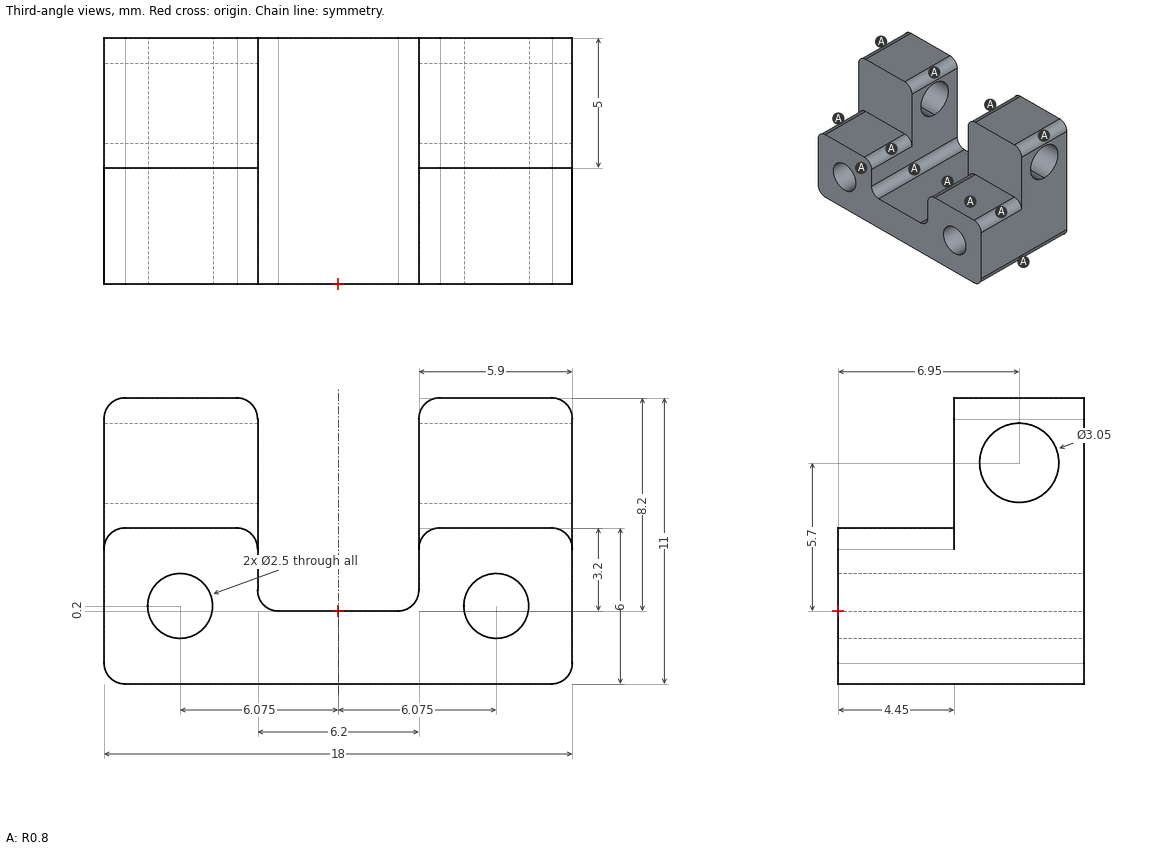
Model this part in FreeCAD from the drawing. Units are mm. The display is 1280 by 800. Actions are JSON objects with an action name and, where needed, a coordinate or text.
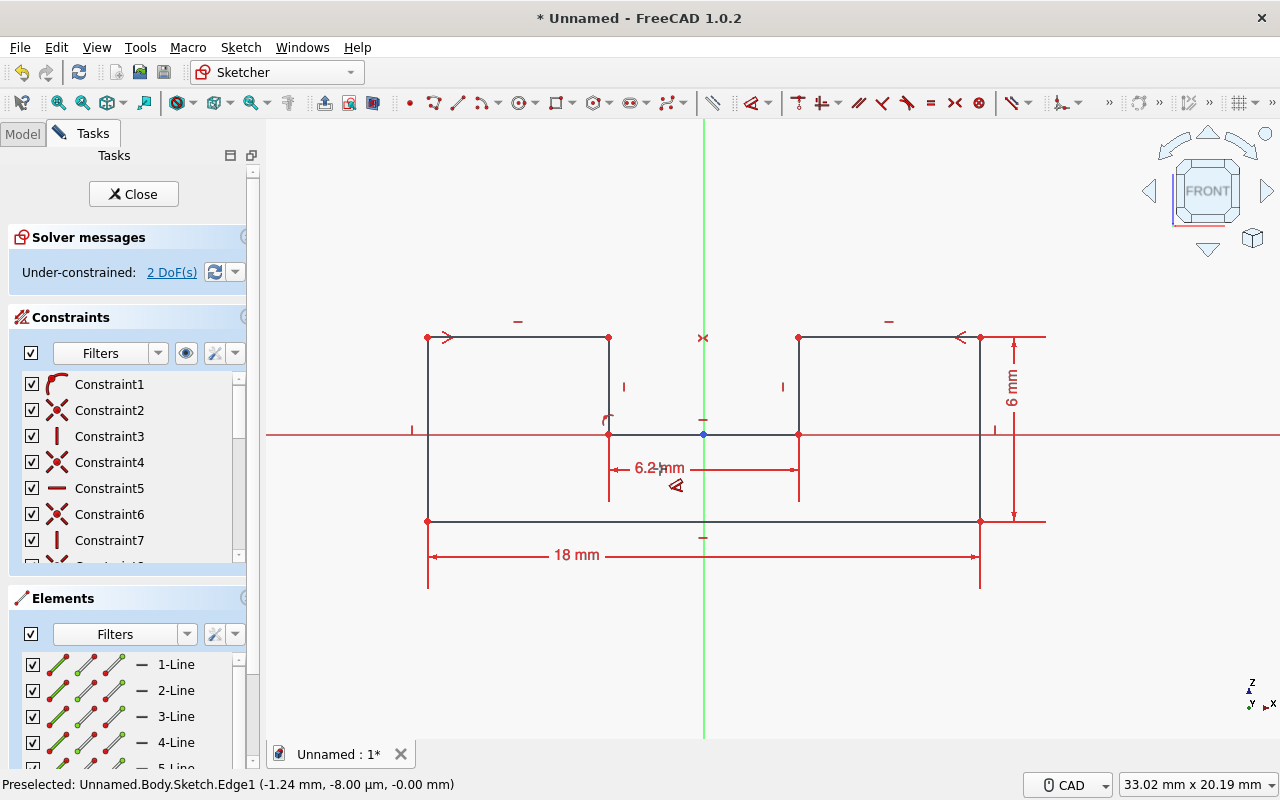
{"action": "left_click", "coordinate": [799, 406]}
{"action": "left_click", "coordinate": [833, 386]}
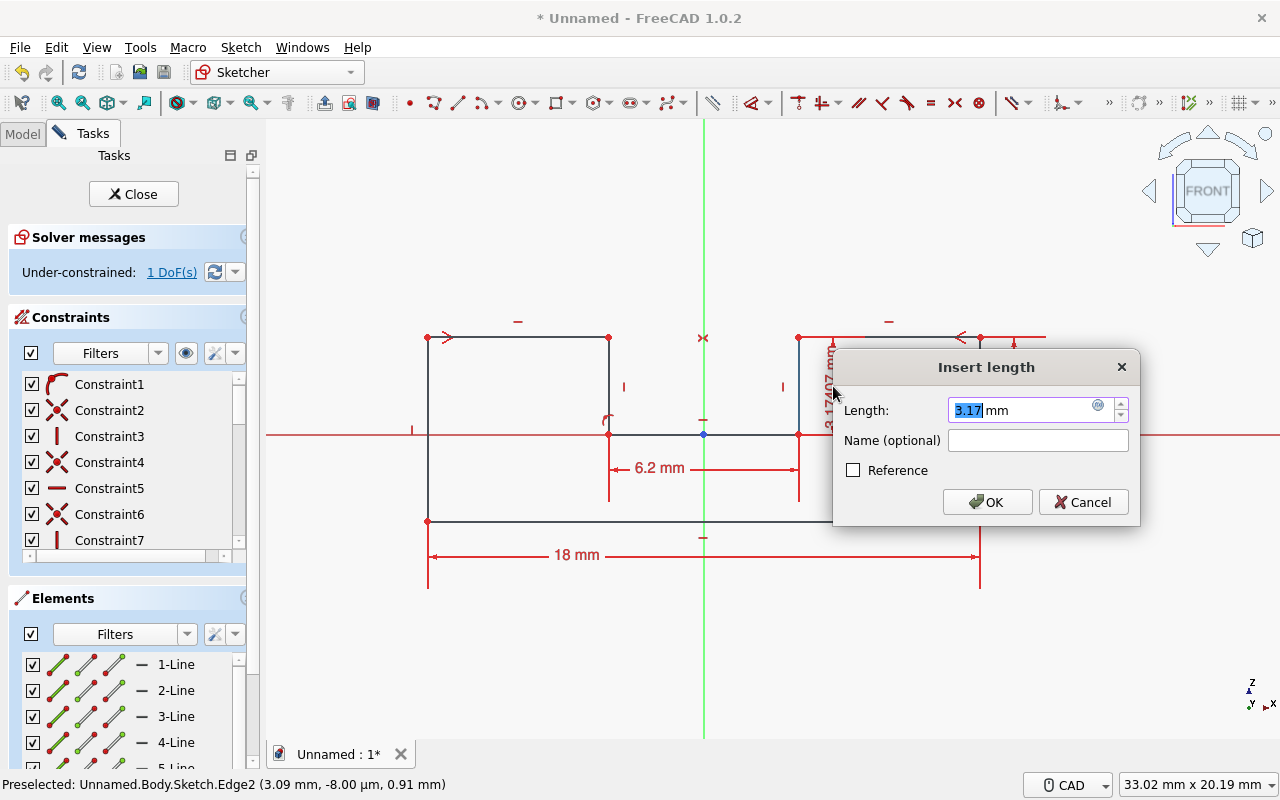
{"action": "type", "text": "3.2"}
{"action": "key", "text": "Return"}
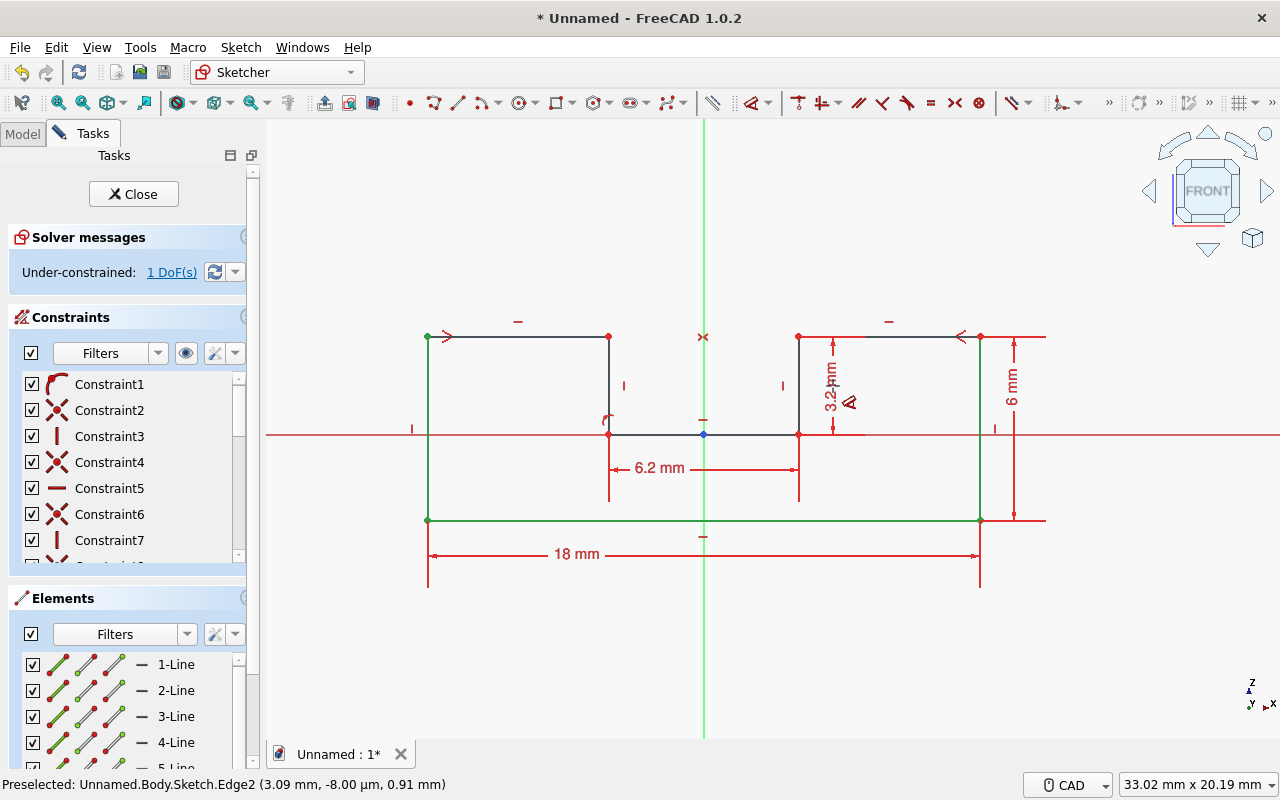
{"action": "left_click", "coordinate": [853, 337]}
{"action": "left_click", "coordinate": [890, 303]}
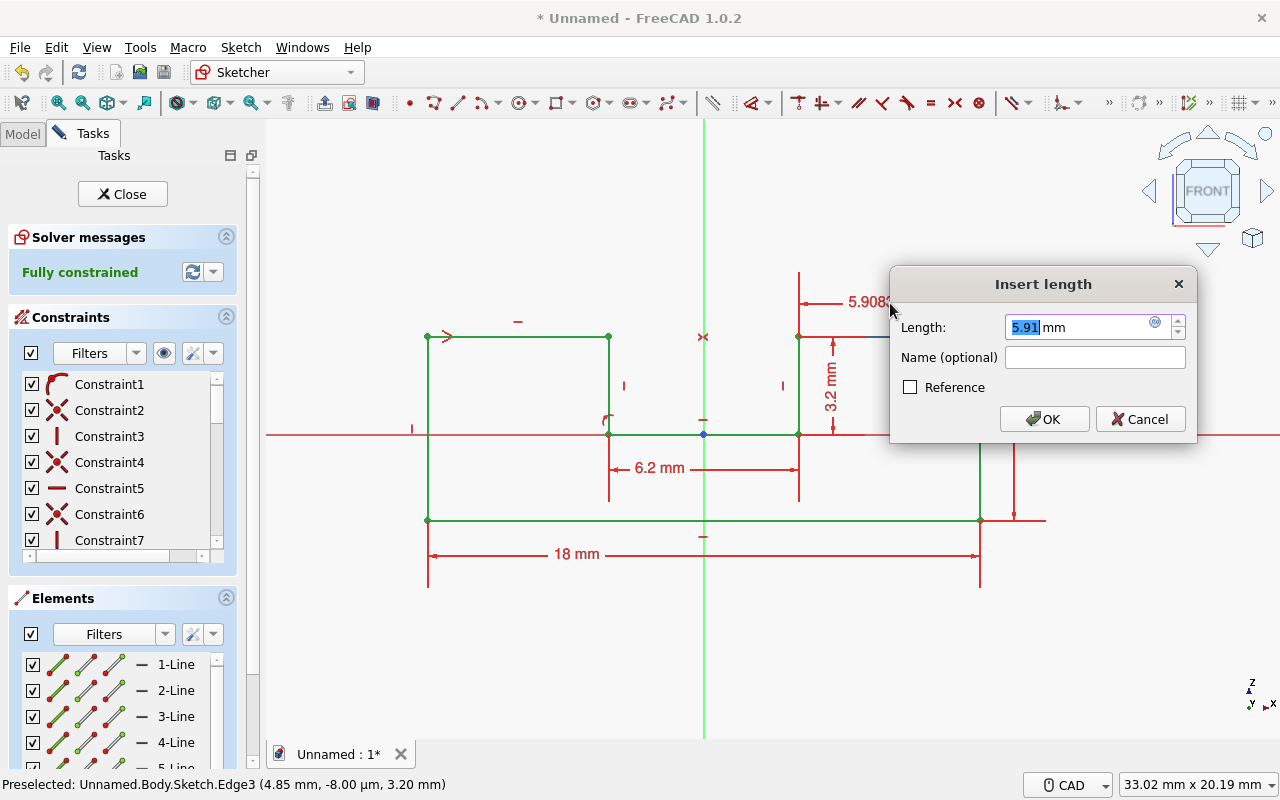
{"action": "type", "text": "5.9"}
{"action": "key", "text": "Return"}
{"action": "key", "text": "Escape"}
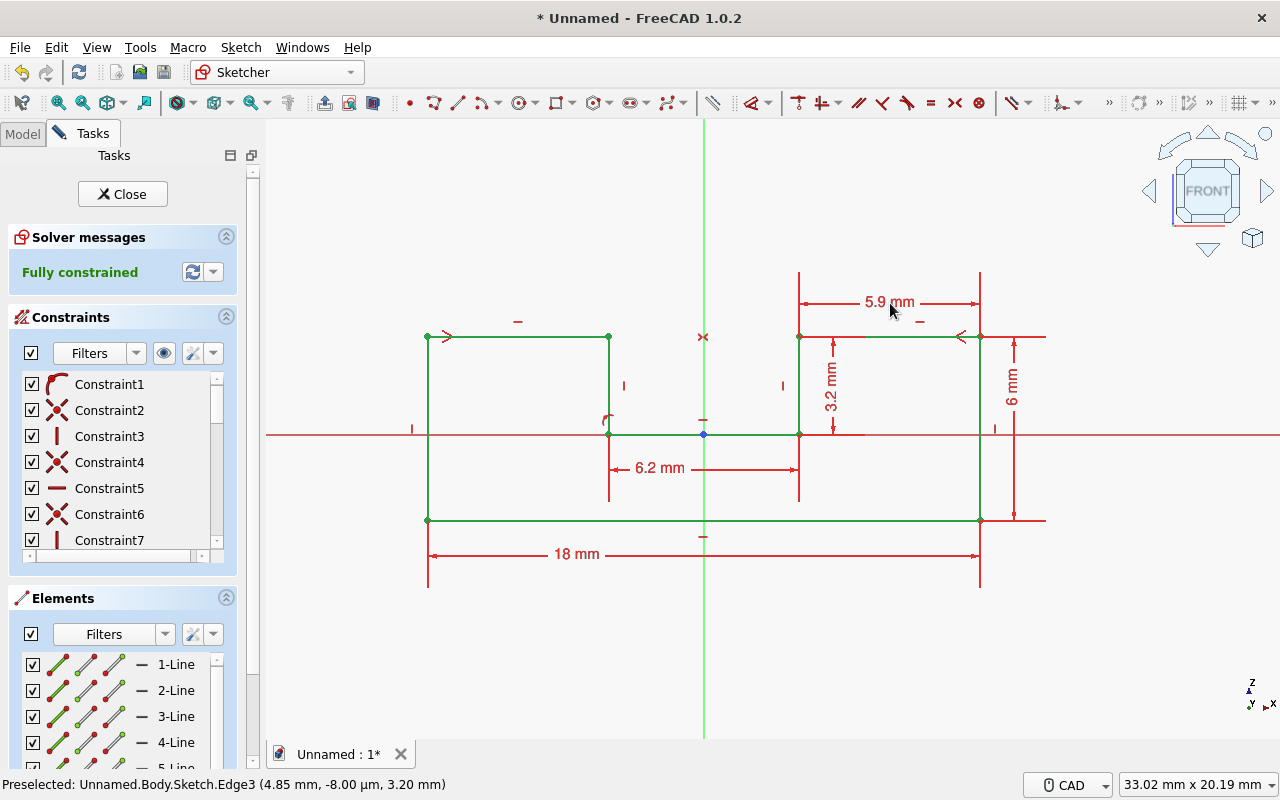
{"action": "left_click", "coordinate": [123, 194]}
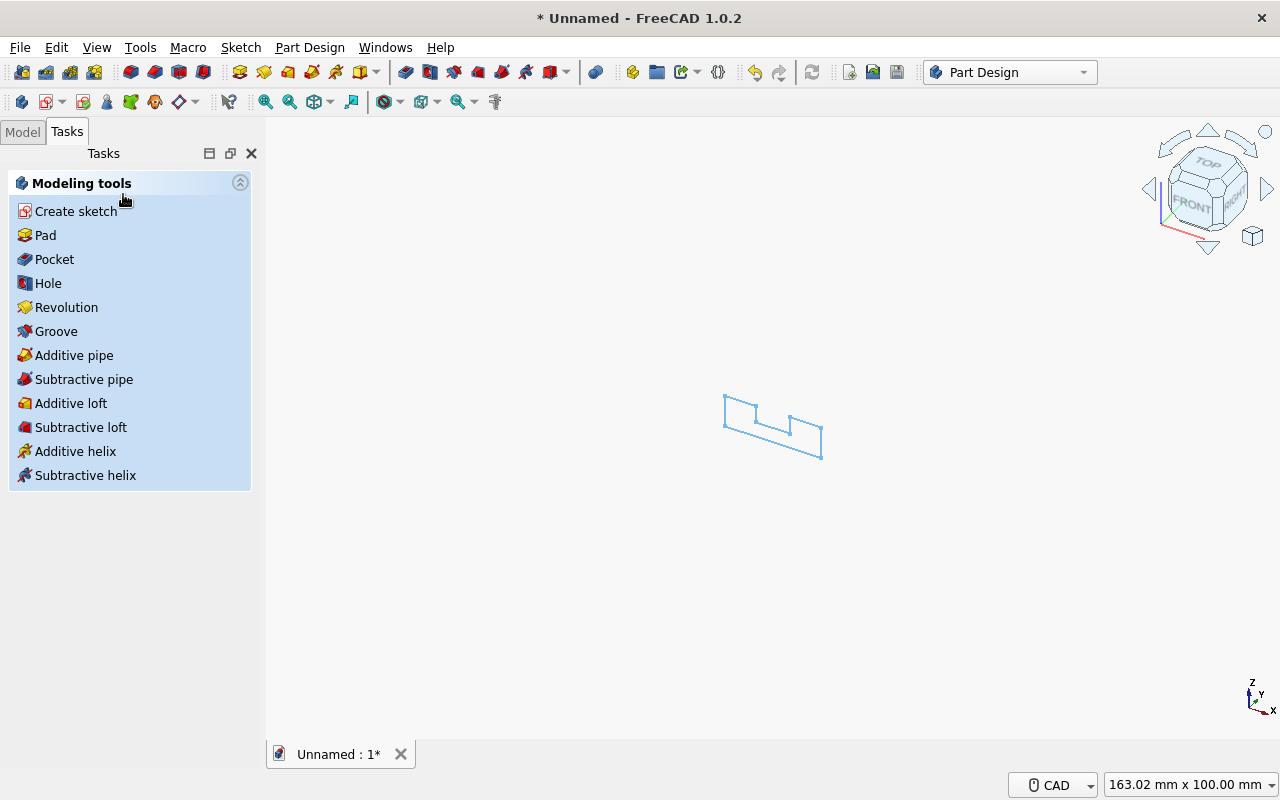
{"action": "left_click", "coordinate": [240, 72]}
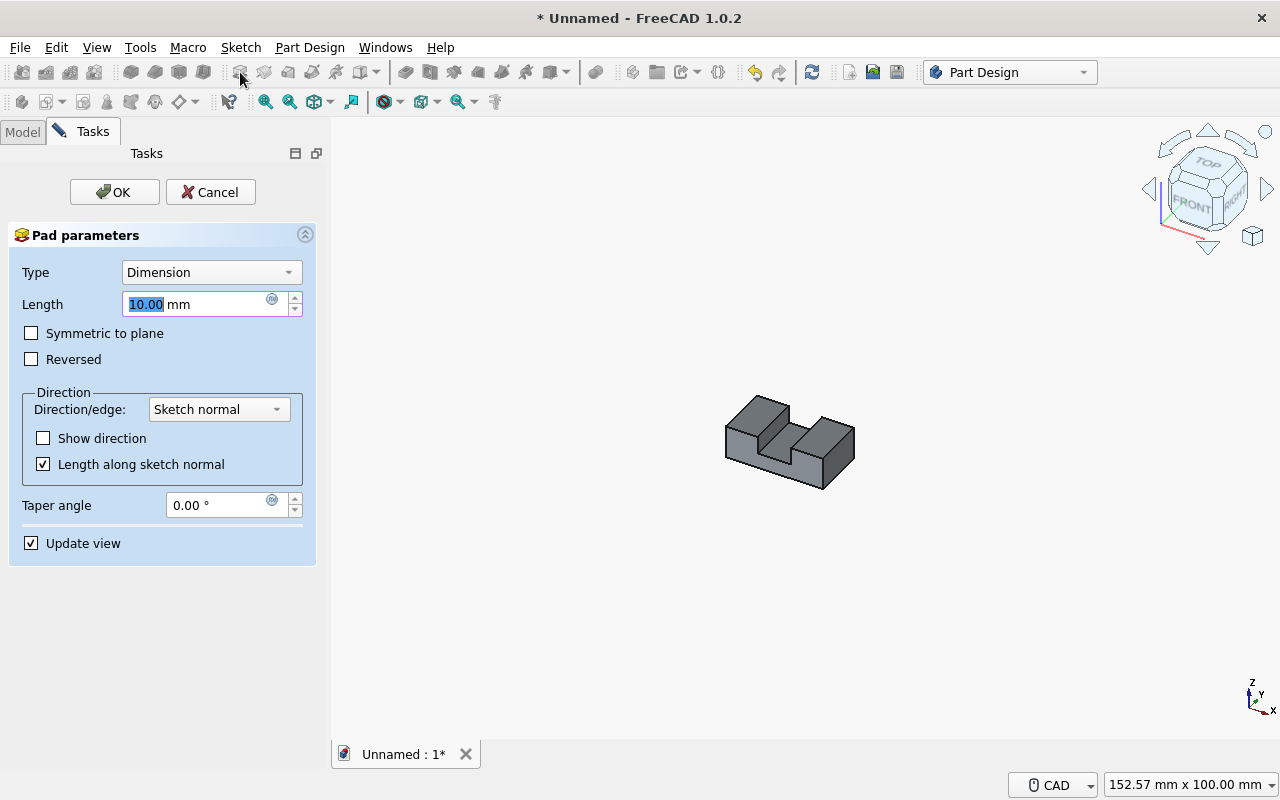
{"action": "type", "text": "4.45"}
{"action": "key", "text": "Tab"}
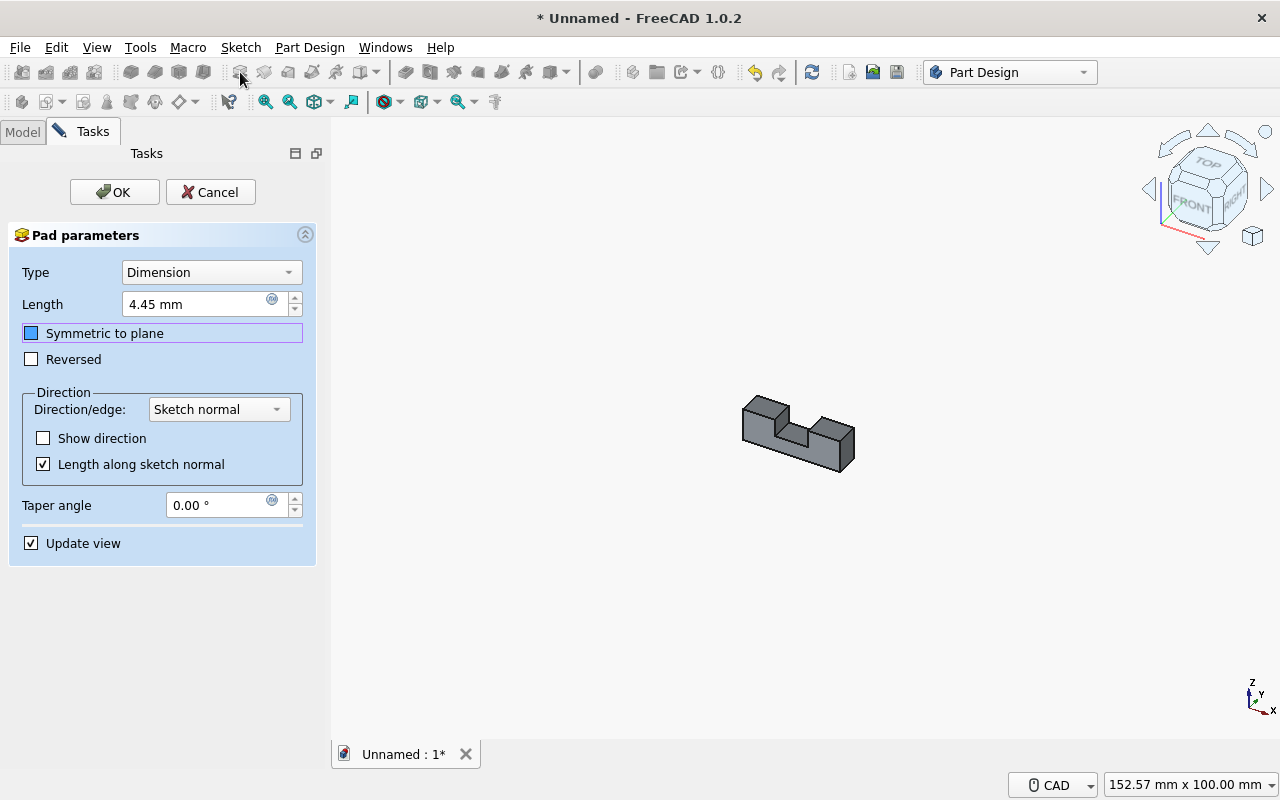
{"action": "left_click", "coordinate": [30, 359]}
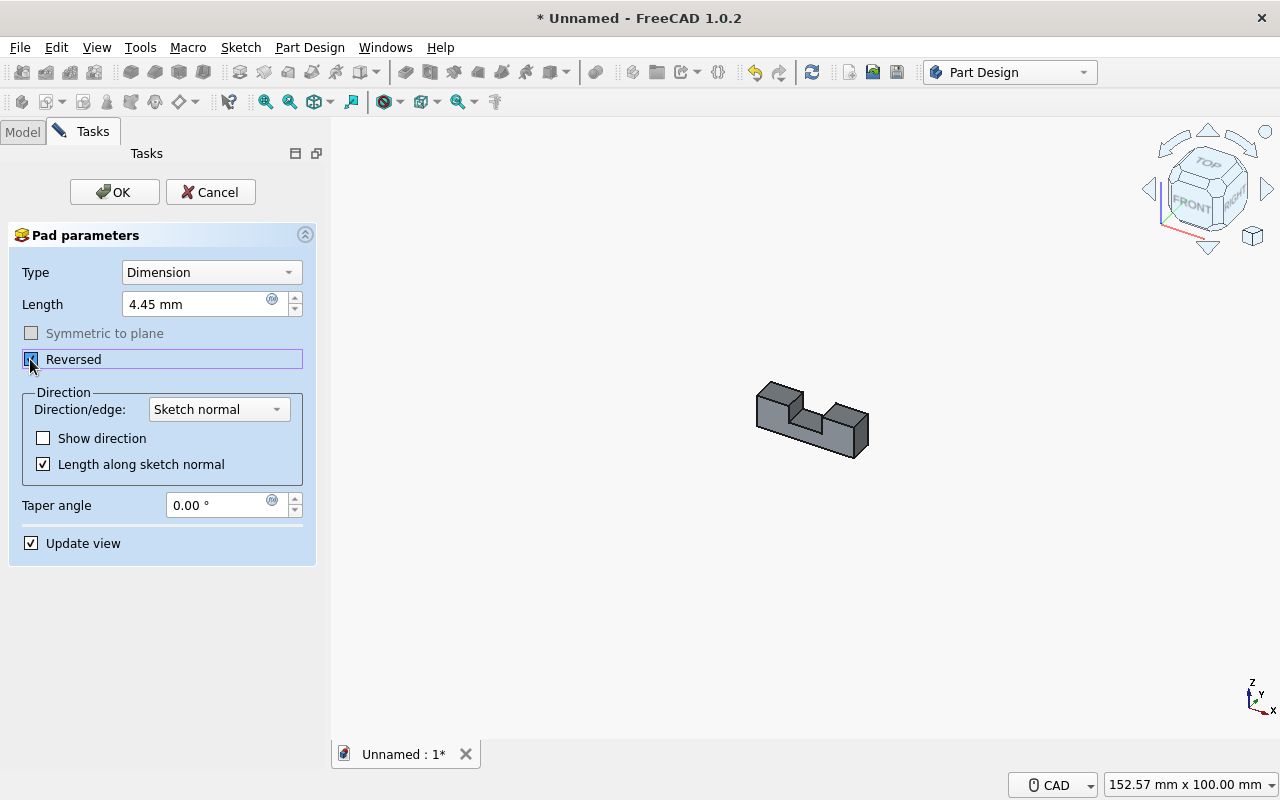
{"action": "left_click", "coordinate": [115, 192]}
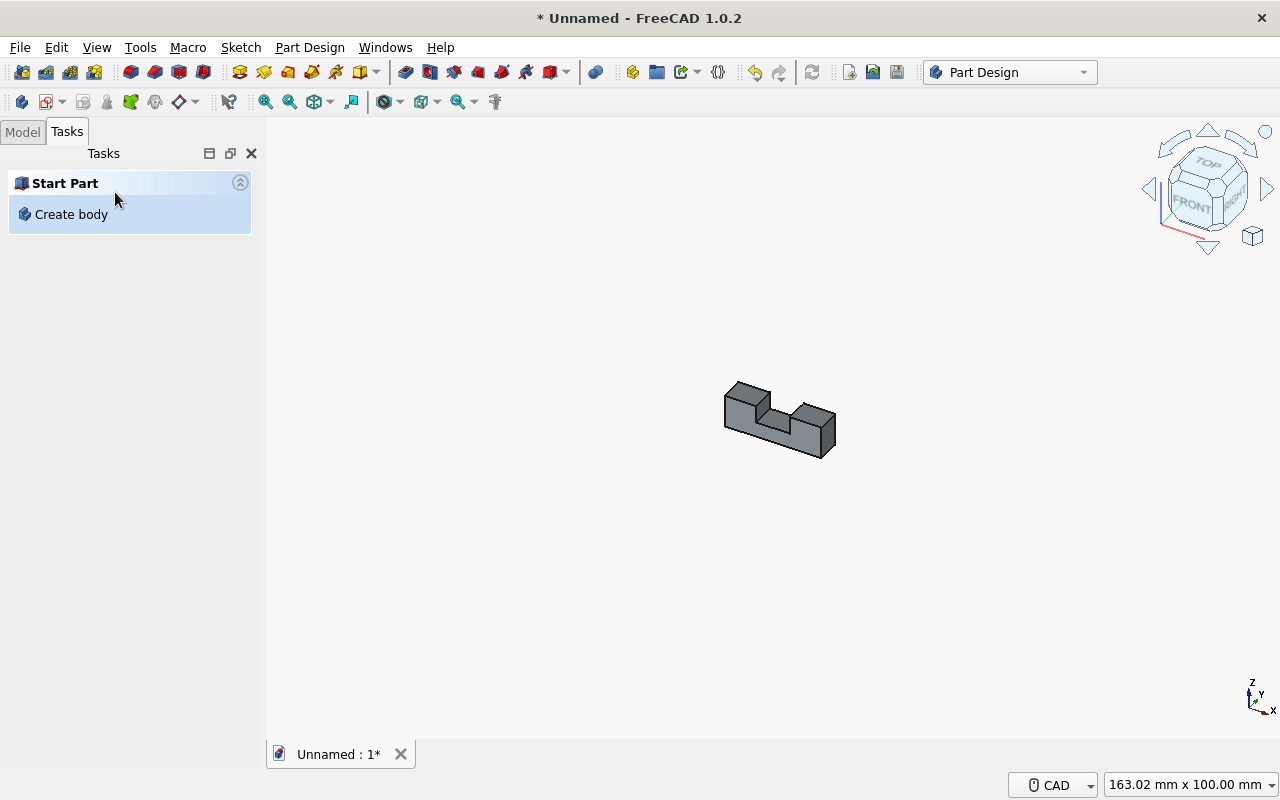
{"action": "left_click", "coordinate": [266, 102]}